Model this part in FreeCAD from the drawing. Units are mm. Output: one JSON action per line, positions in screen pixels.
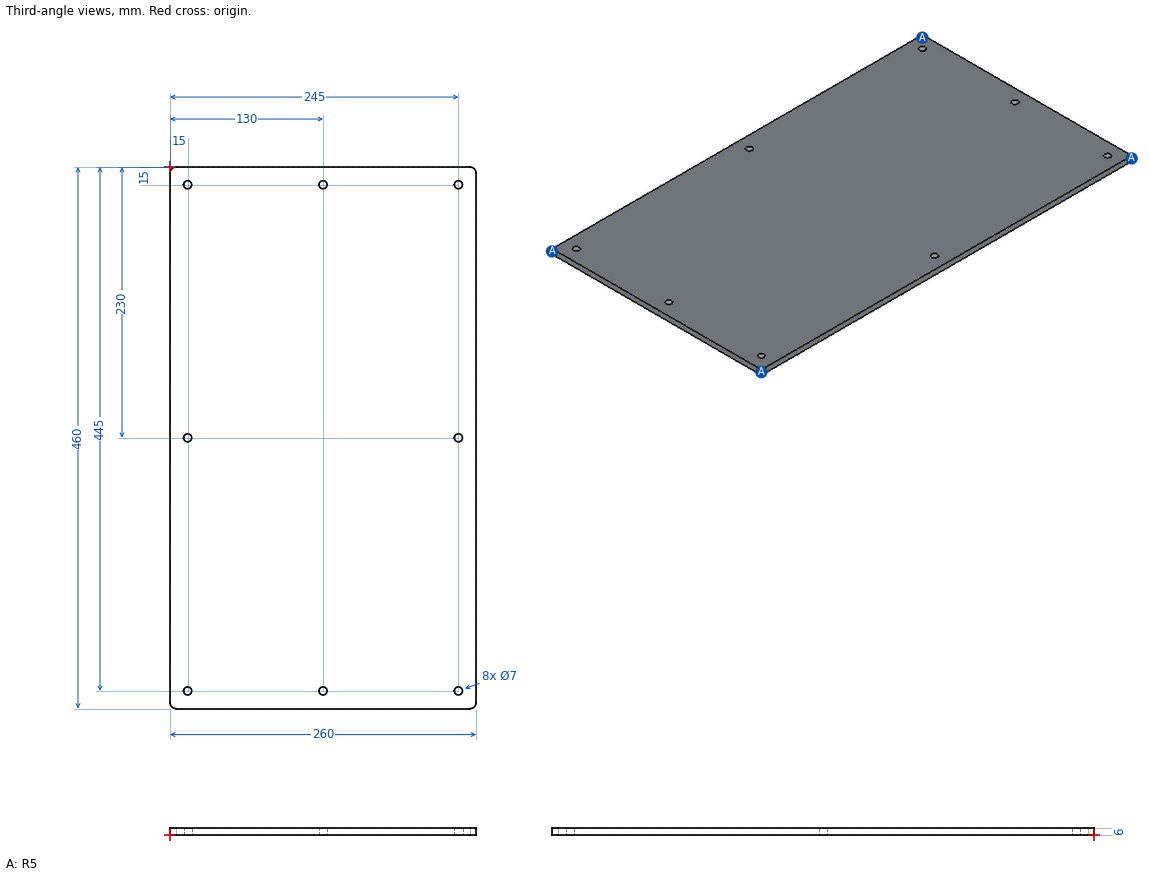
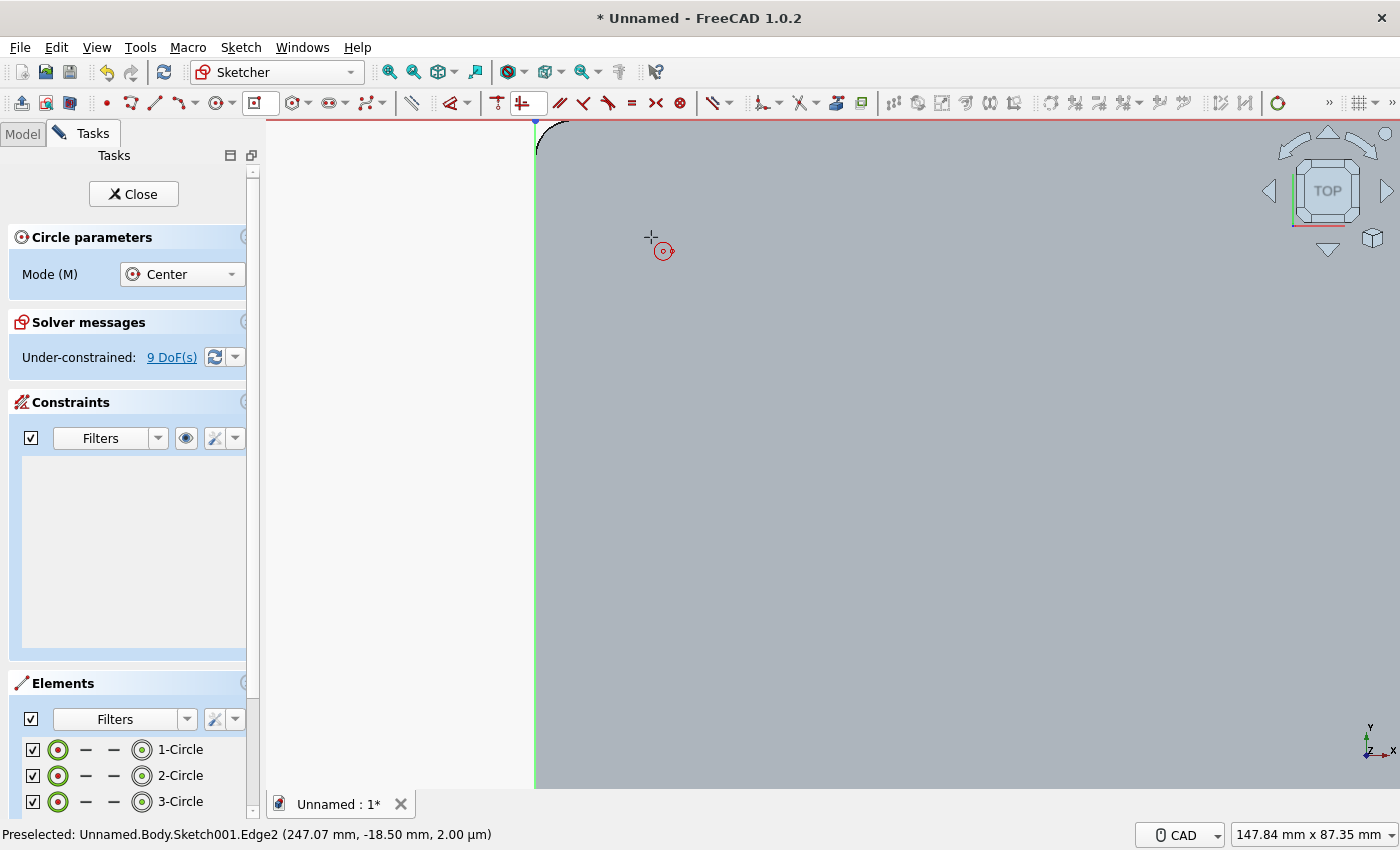
{"action": "scroll", "coordinate": [651, 237], "scroll_direction": "down", "scroll_amount": 10}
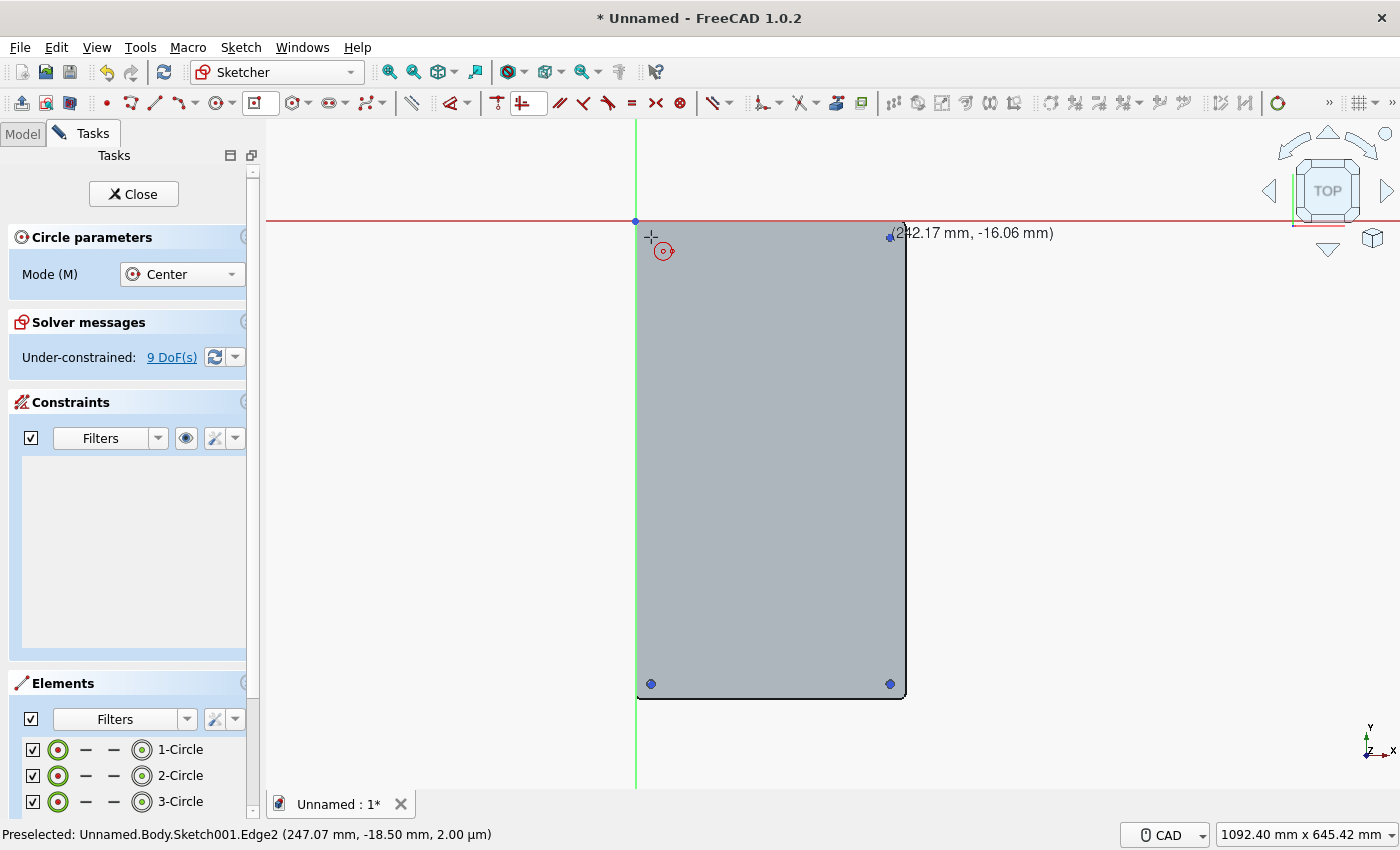
{"action": "left_click", "coordinate": [651, 237]}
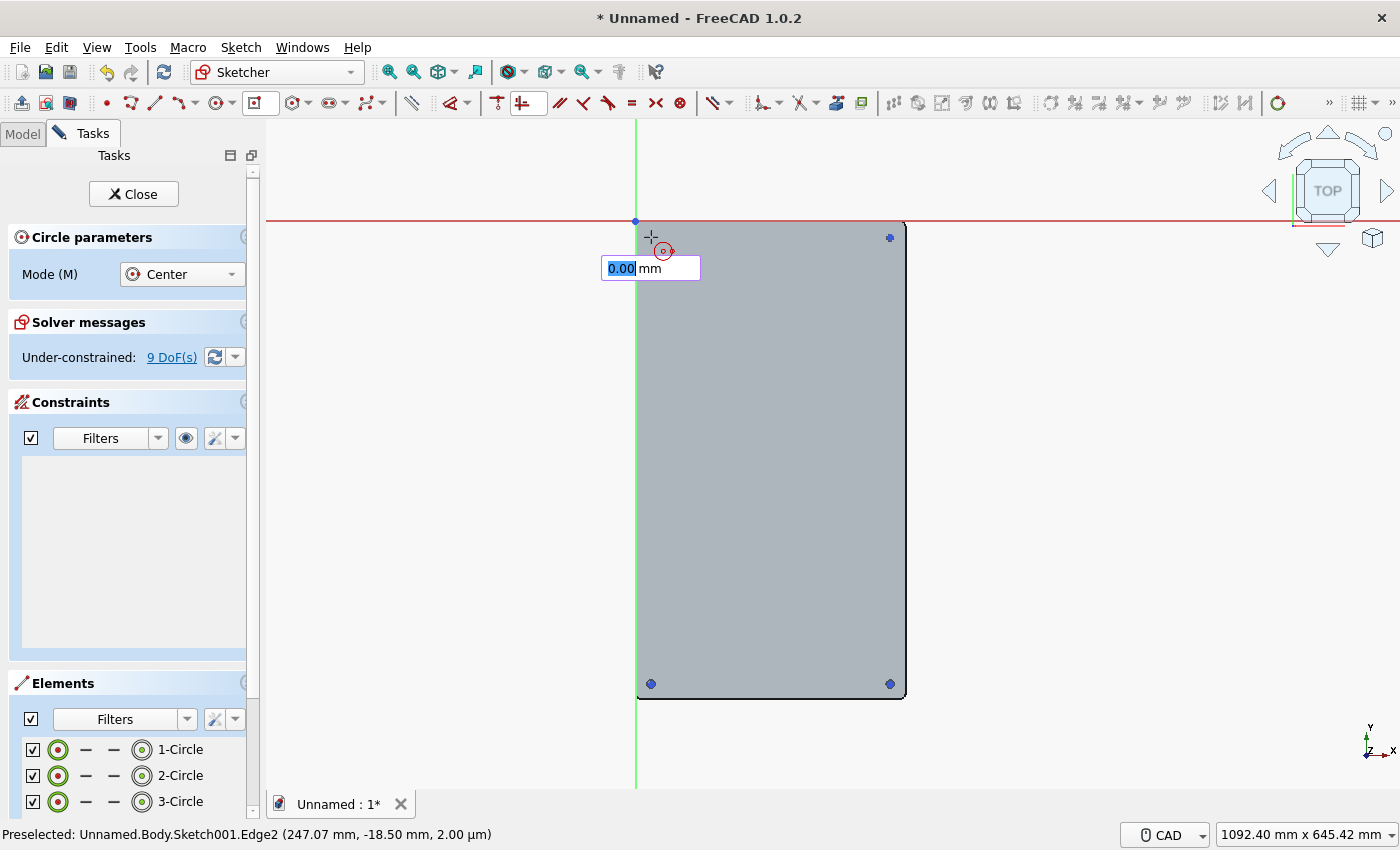
{"action": "scroll", "coordinate": [654, 239], "scroll_direction": "up", "scroll_amount": 8}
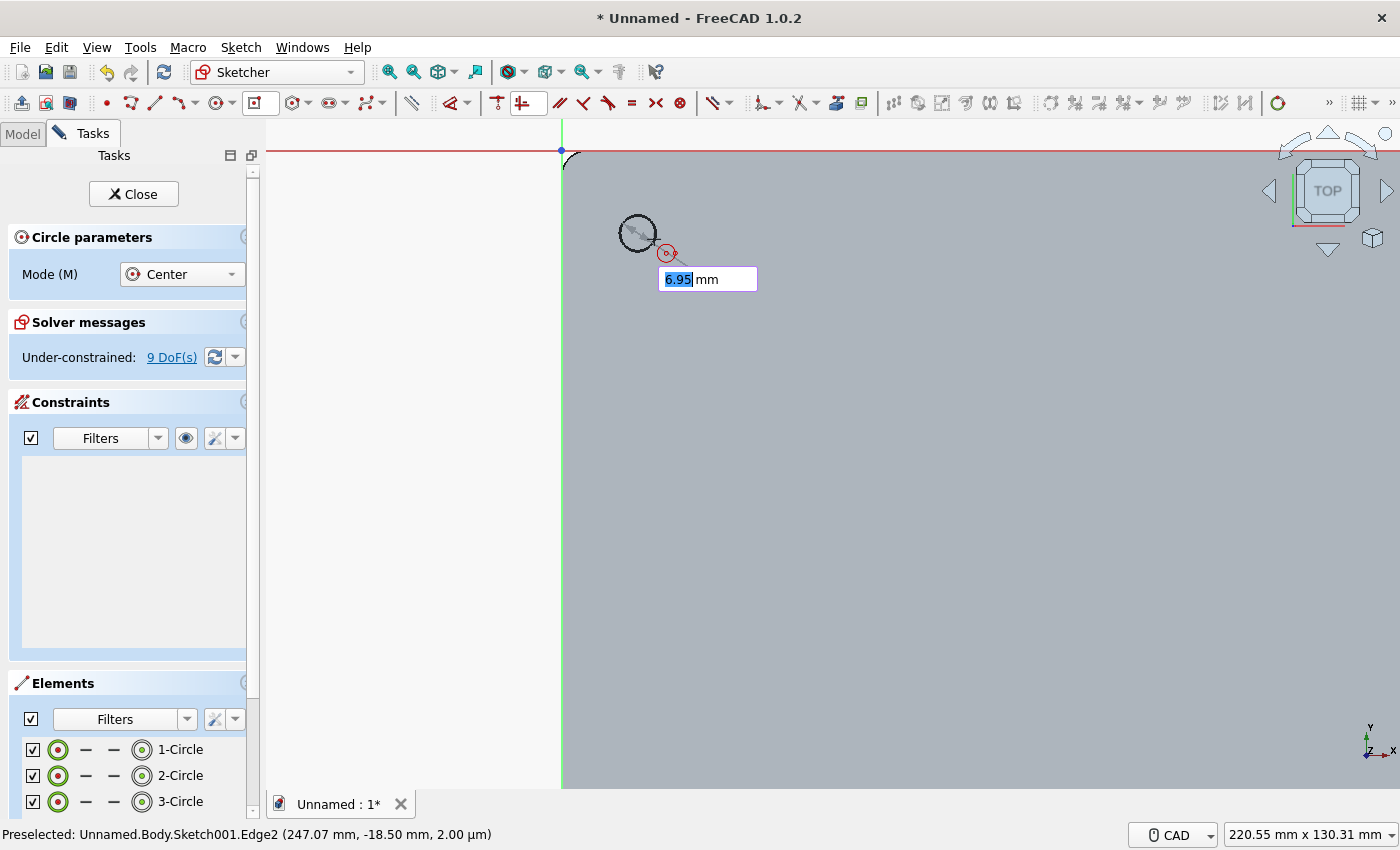
{"action": "left_click", "coordinate": [651, 241]}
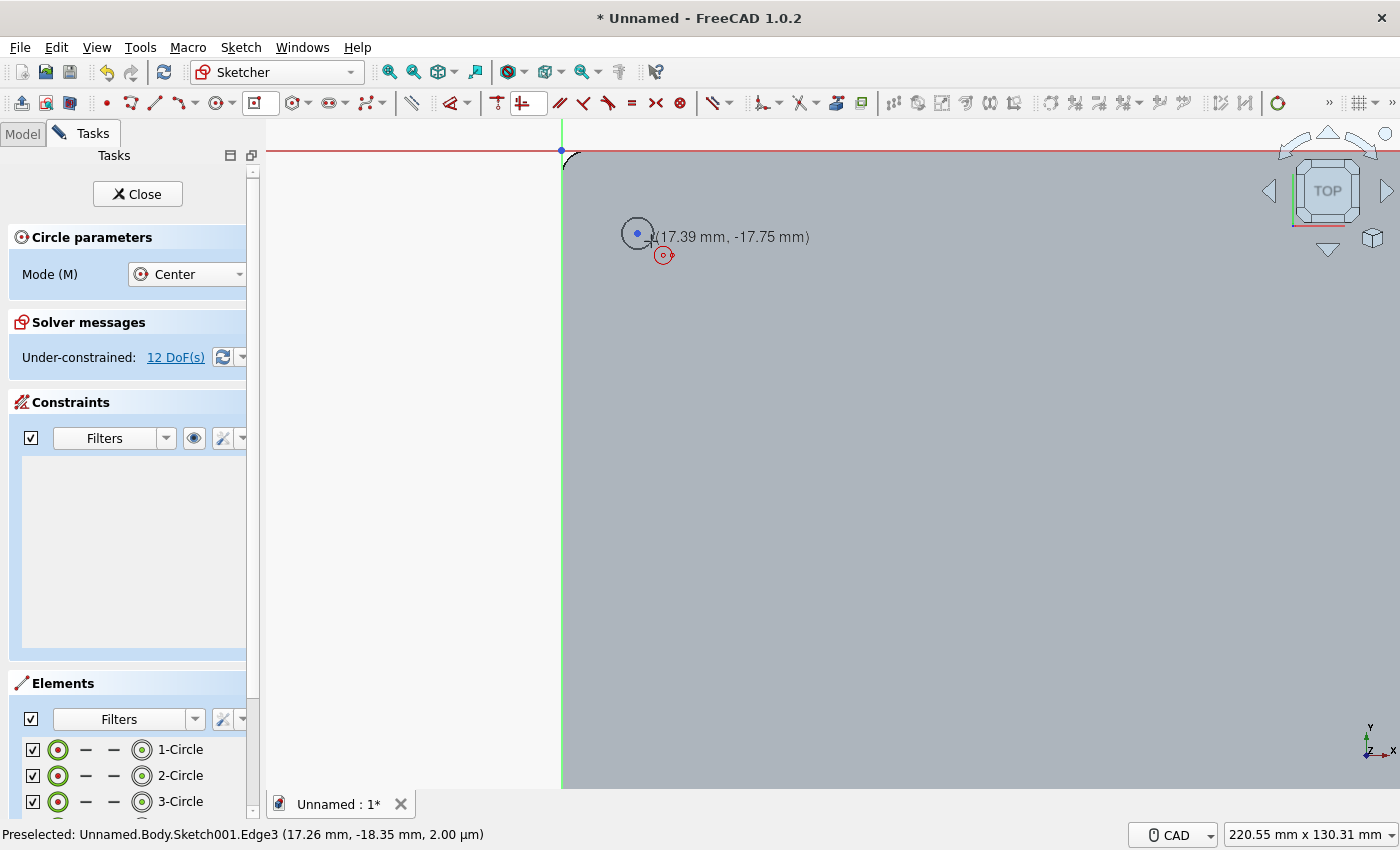
{"action": "scroll", "coordinate": [654, 239], "scroll_direction": "down", "scroll_amount": 8}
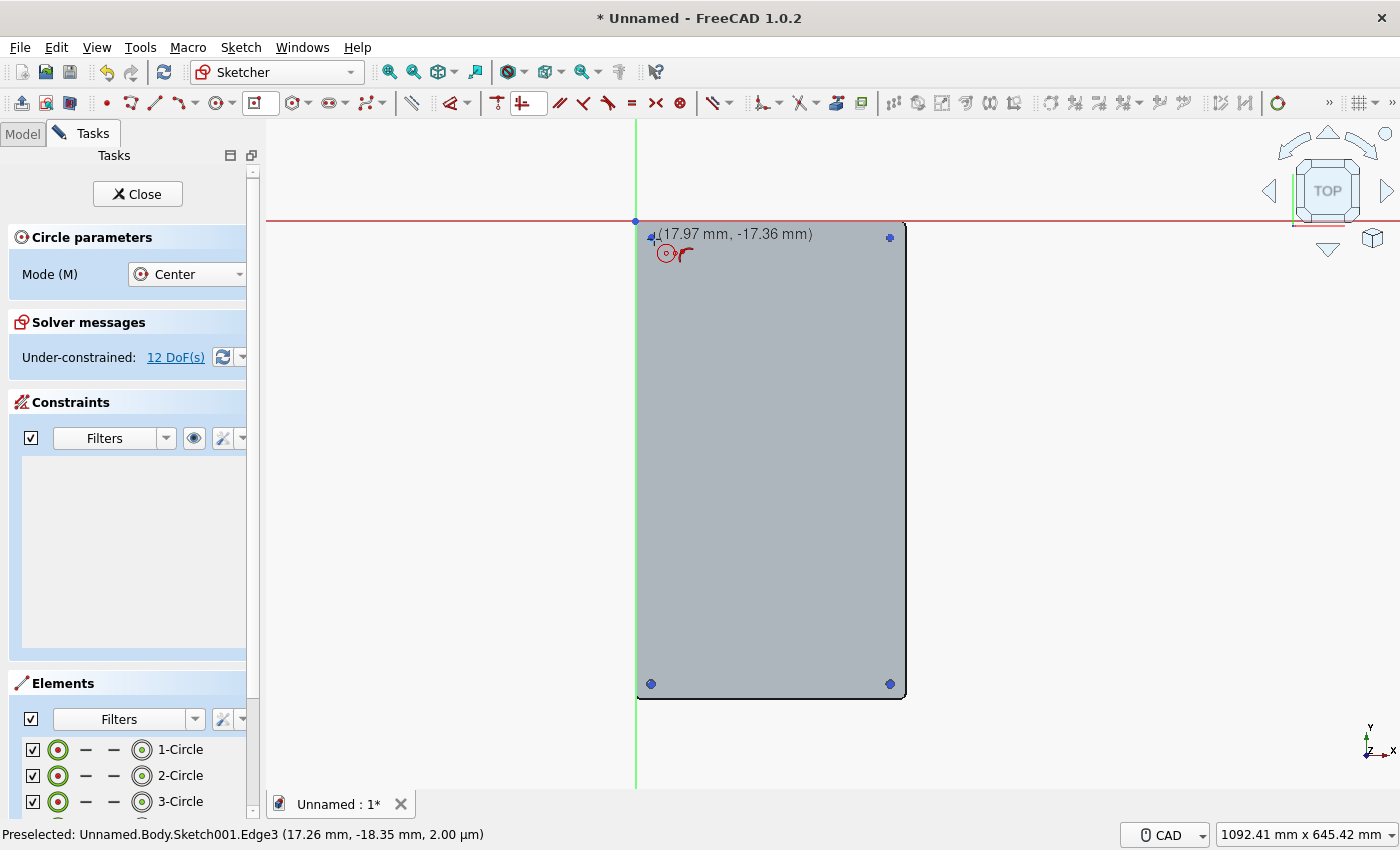
{"action": "scroll", "coordinate": [771, 683], "scroll_direction": "up", "scroll_amount": 10}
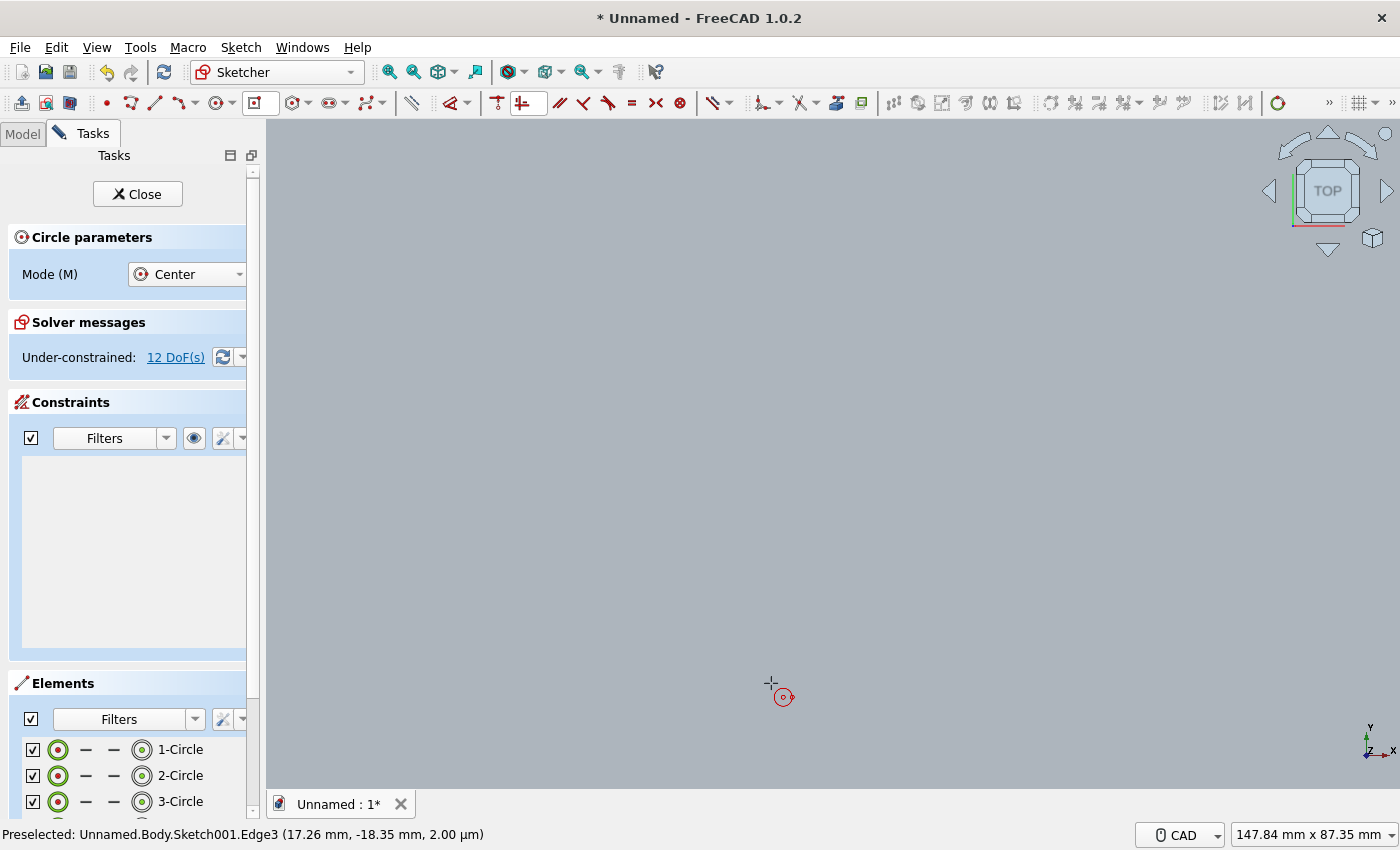
{"action": "scroll", "coordinate": [771, 684], "scroll_direction": "down", "scroll_amount": 10}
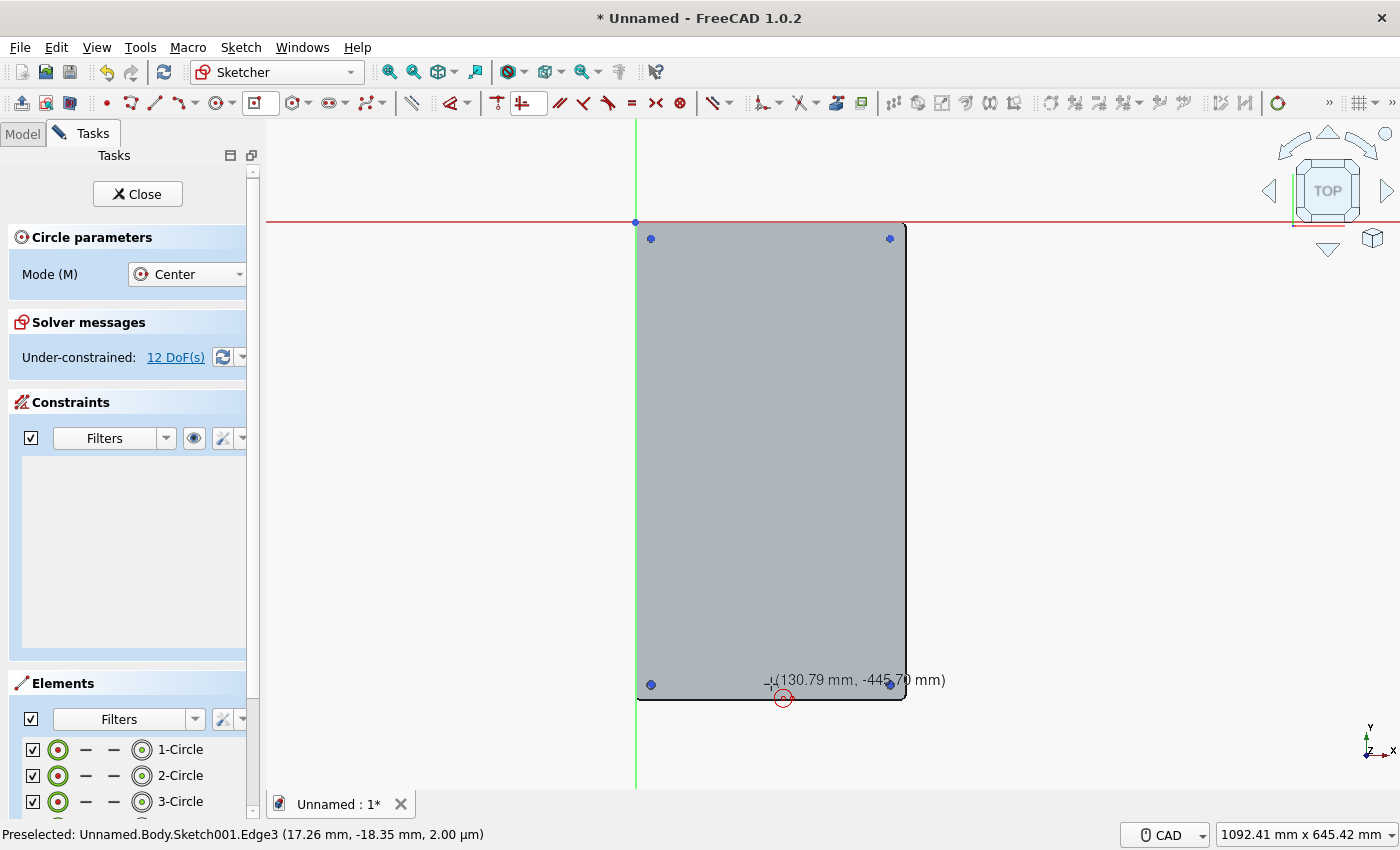
{"action": "left_click", "coordinate": [771, 684]}